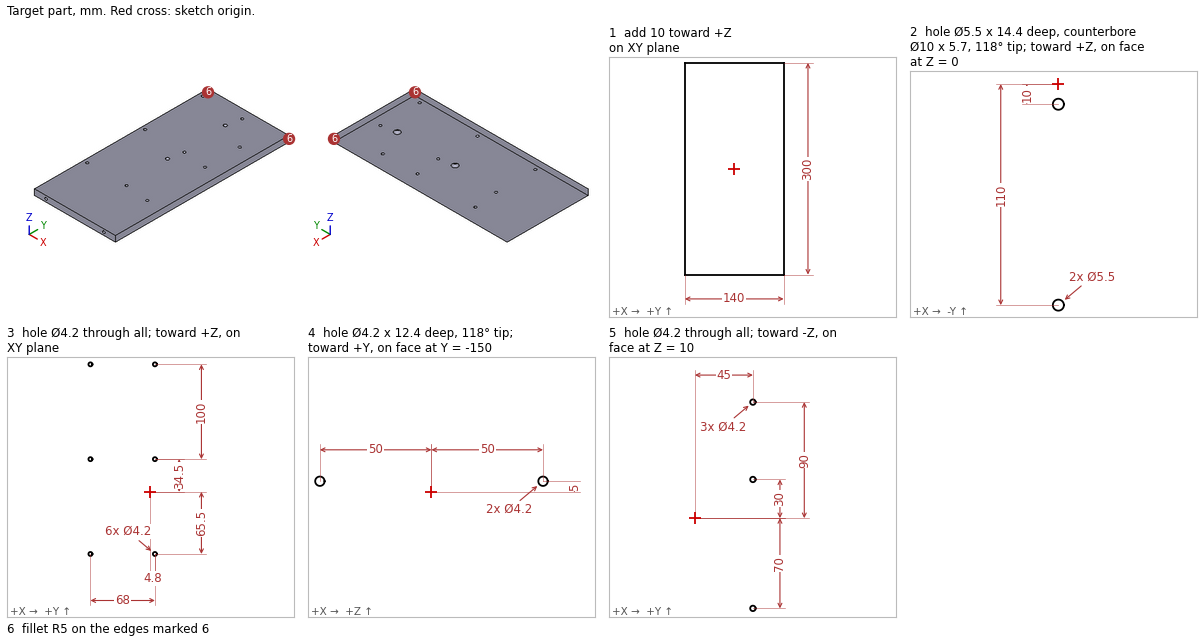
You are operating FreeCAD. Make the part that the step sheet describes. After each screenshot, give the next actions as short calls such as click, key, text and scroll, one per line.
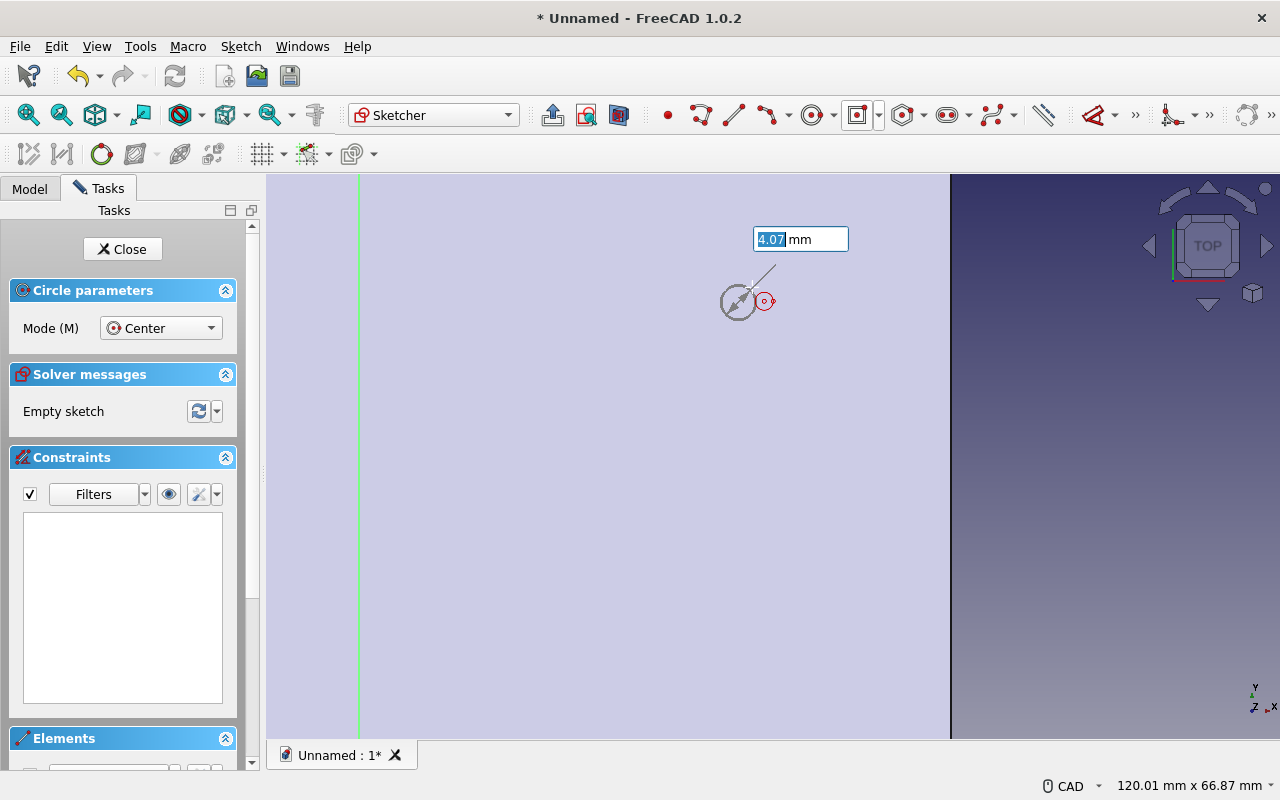
click(752, 288)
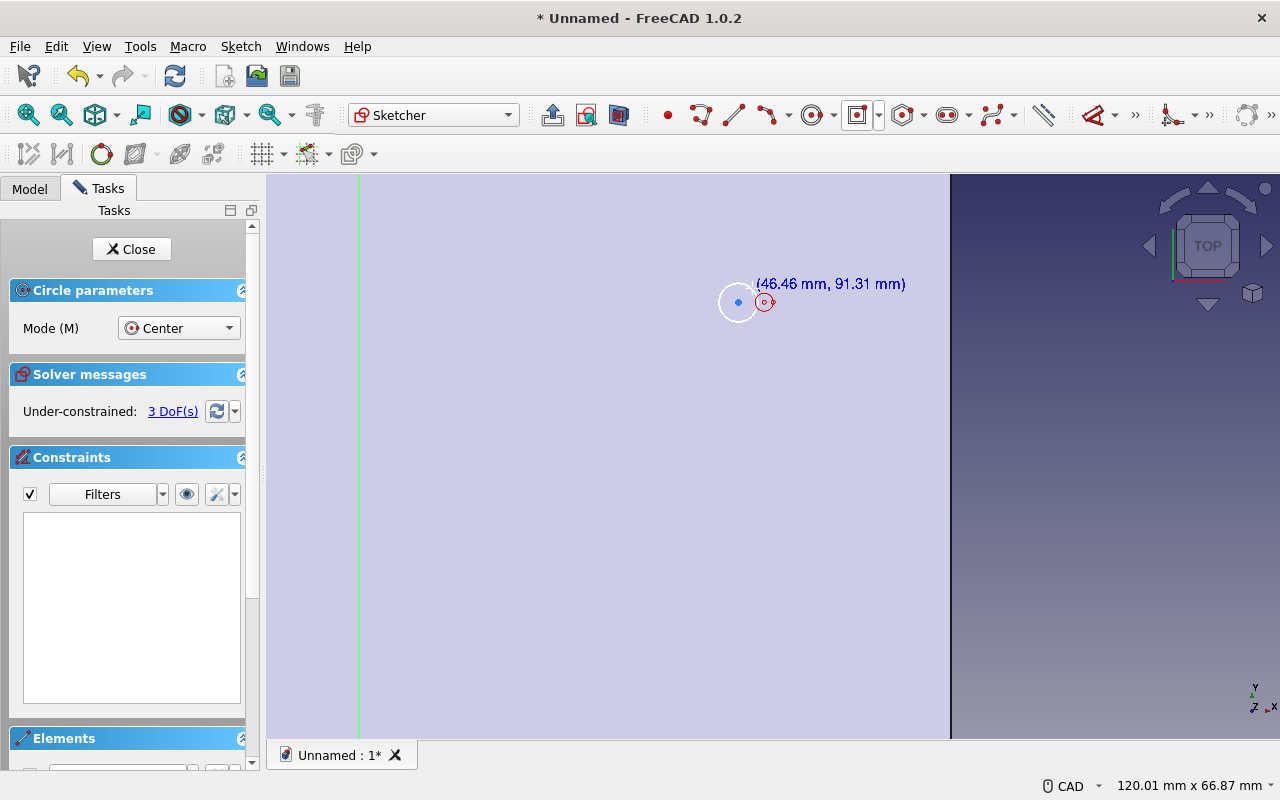
scroll(752, 286, down, 7)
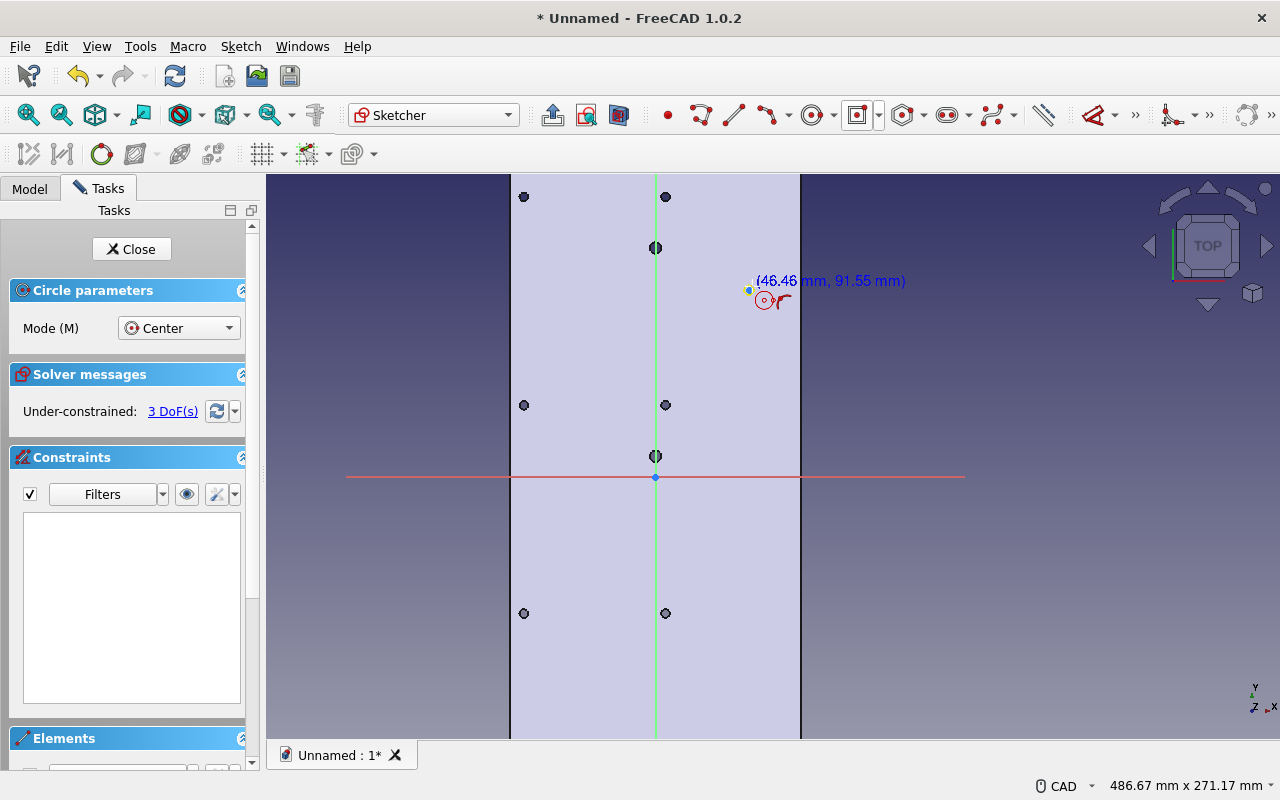
scroll(749, 415, up, 9)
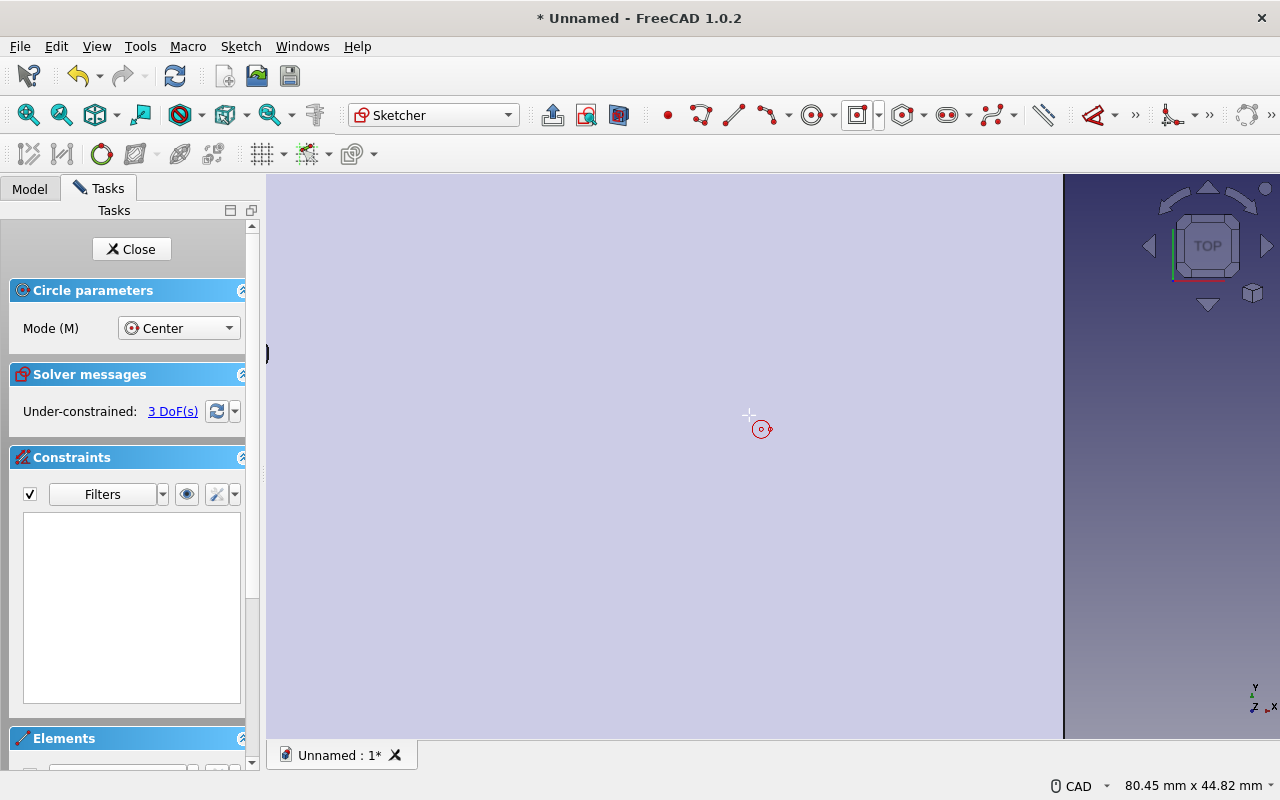
scroll(749, 416, down, 9)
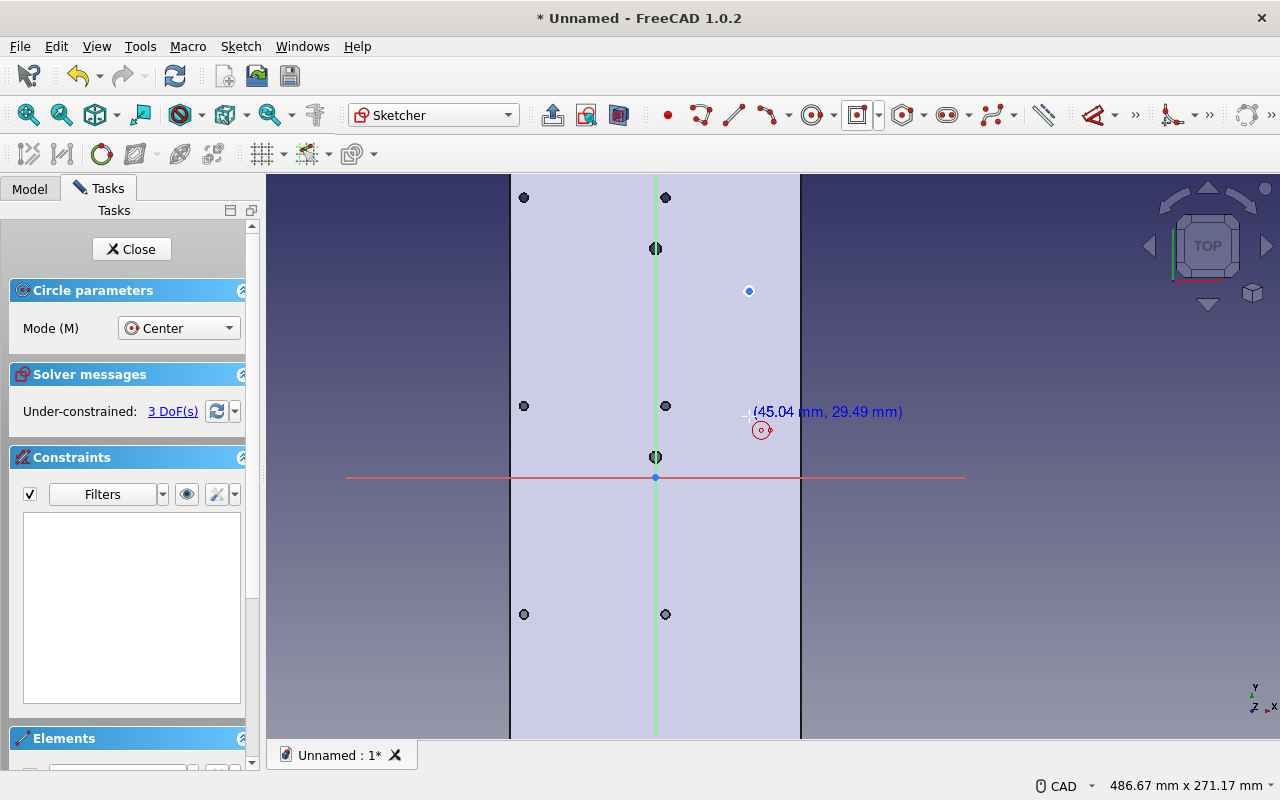
click(749, 415)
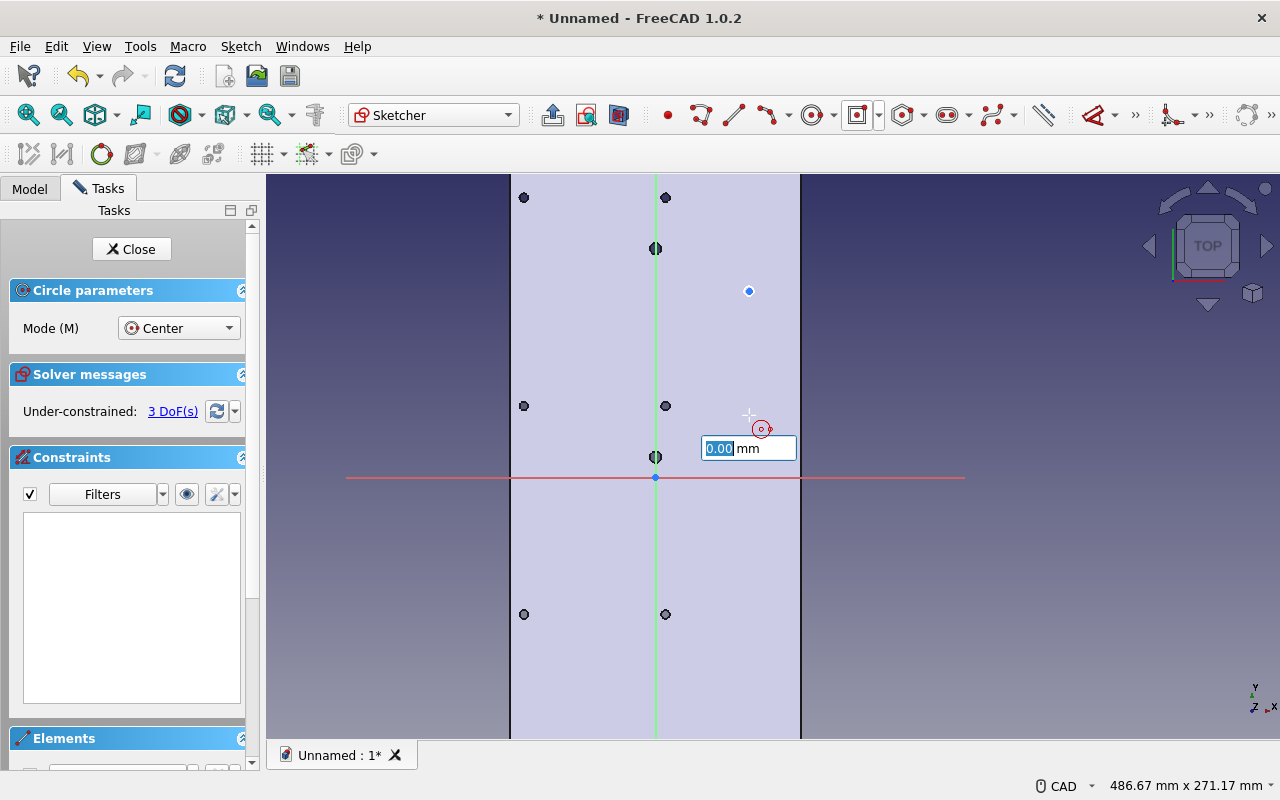
scroll(752, 412, up, 7)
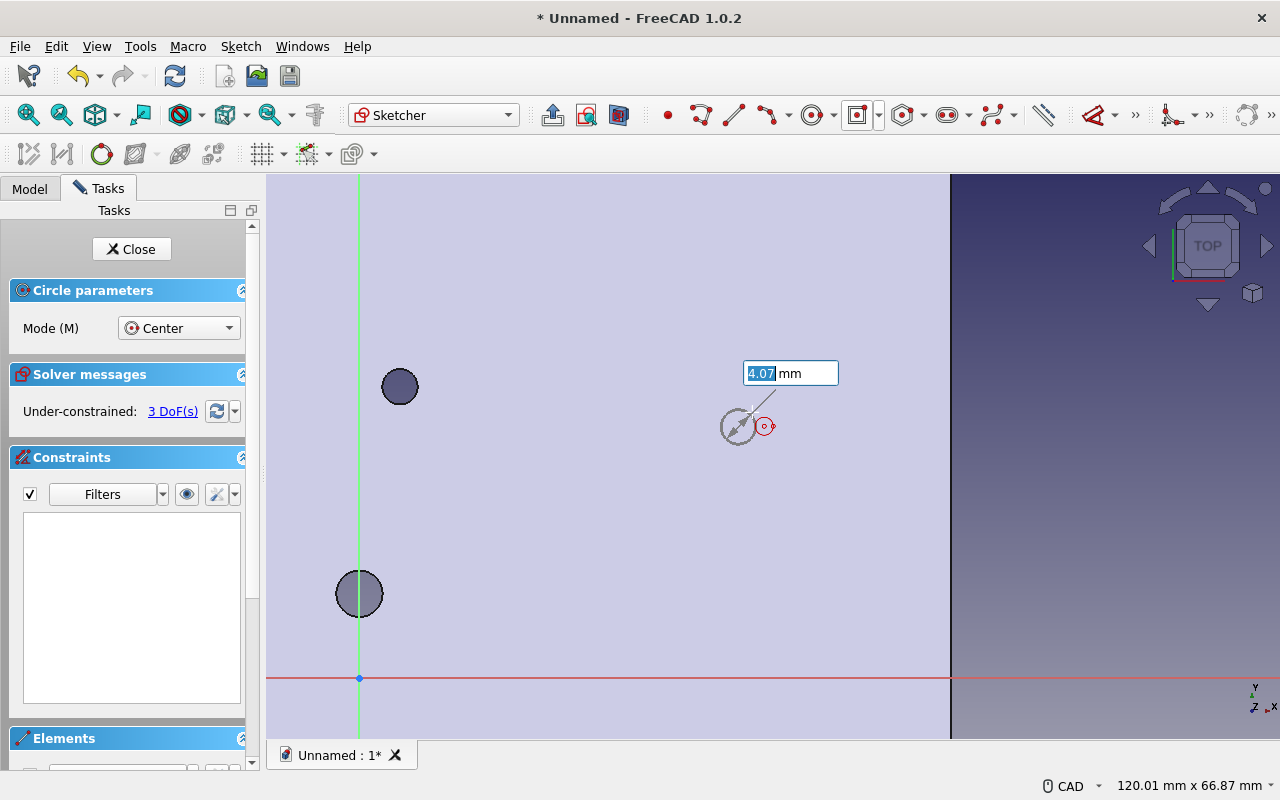
click(752, 412)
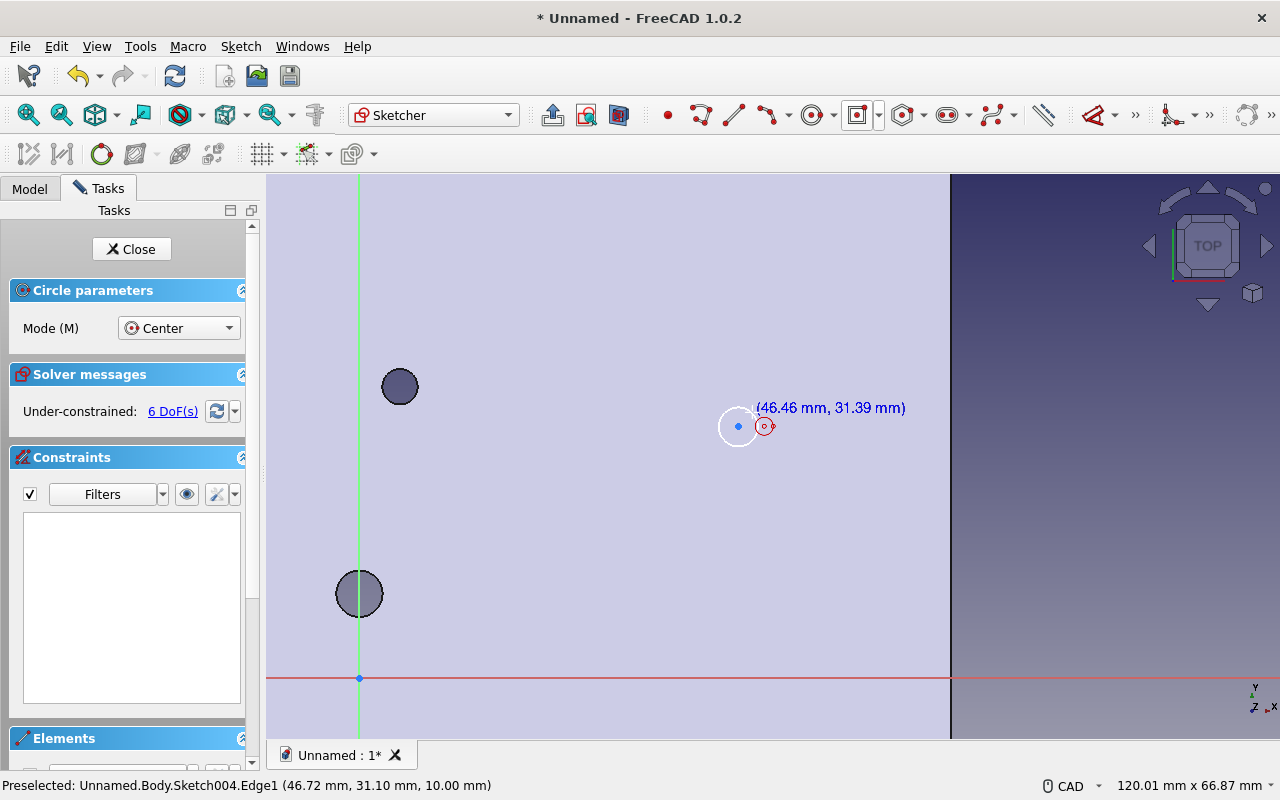
scroll(752, 412, down, 7)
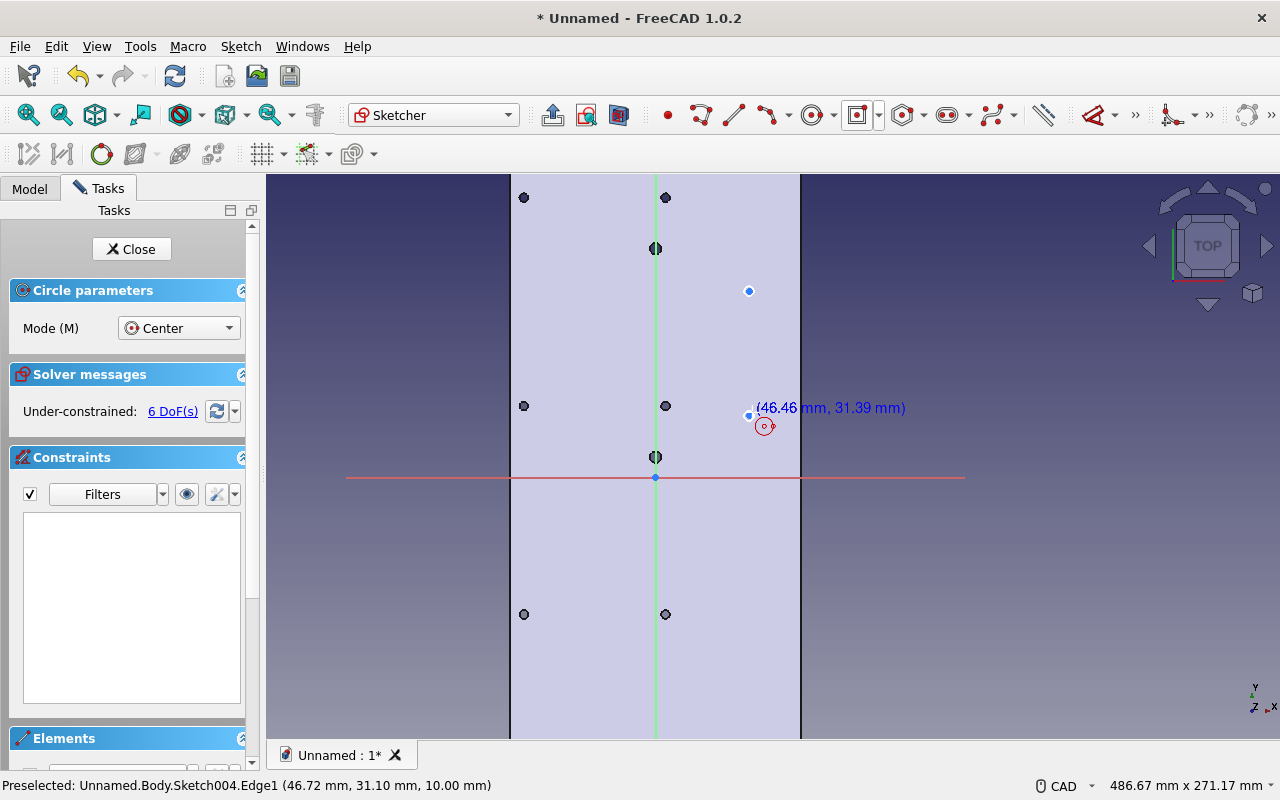
scroll(749, 624, up, 9)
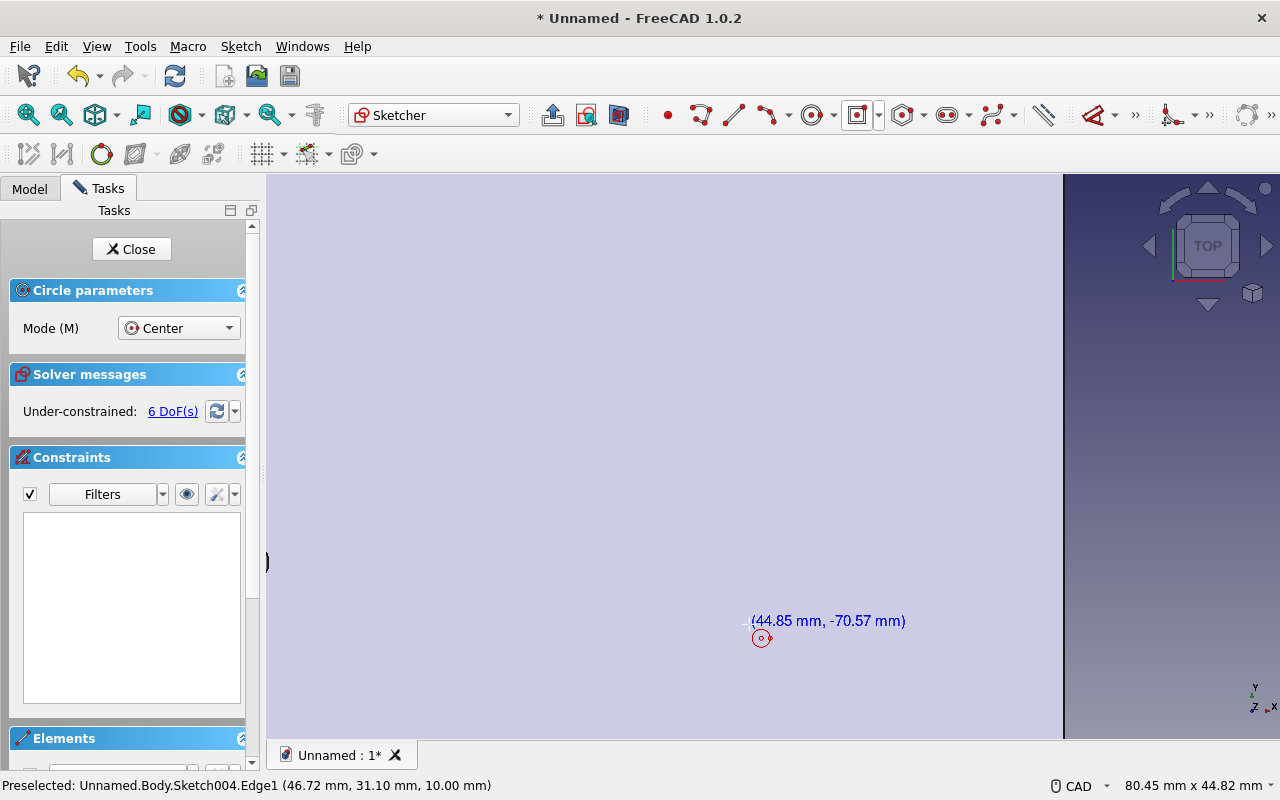
scroll(749, 624, down, 9)